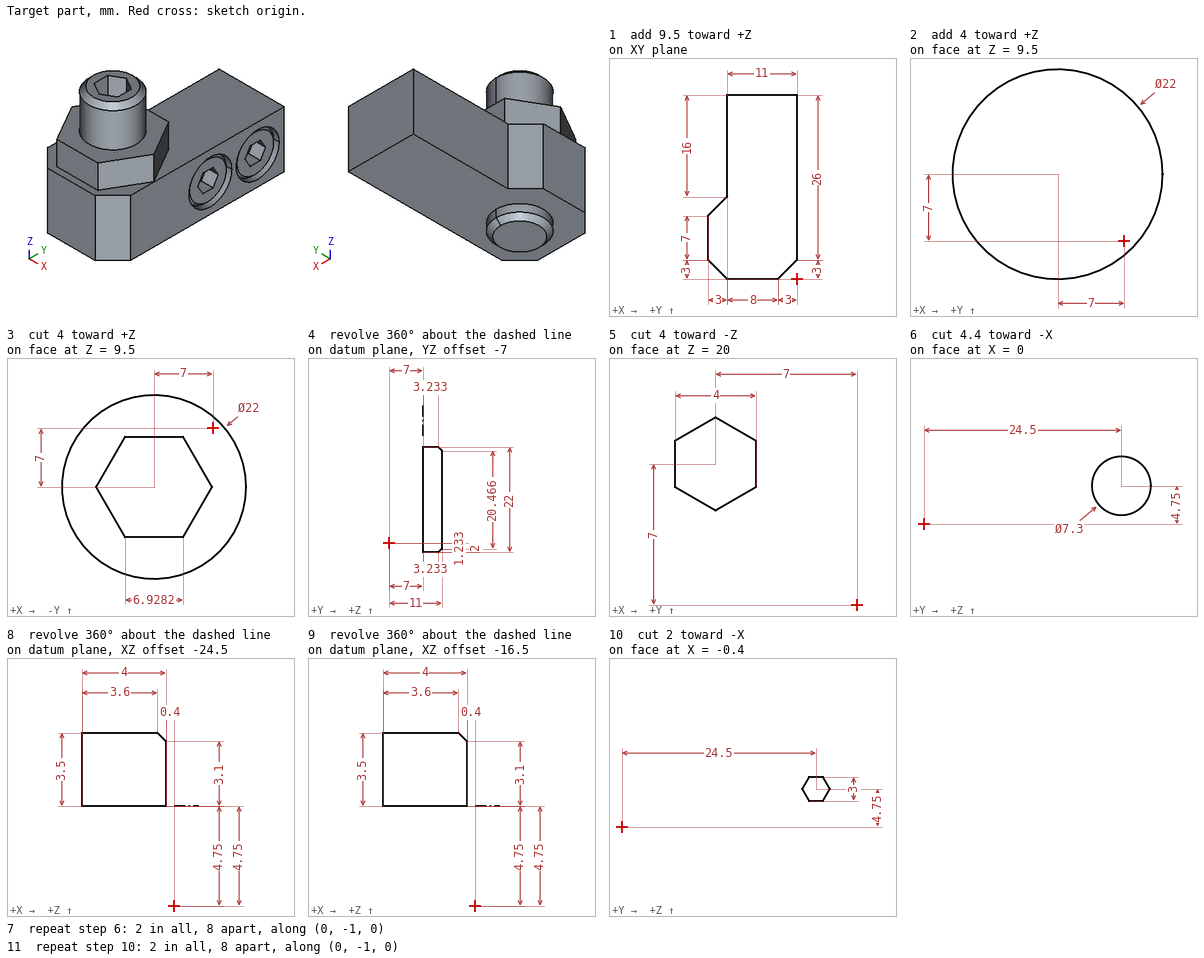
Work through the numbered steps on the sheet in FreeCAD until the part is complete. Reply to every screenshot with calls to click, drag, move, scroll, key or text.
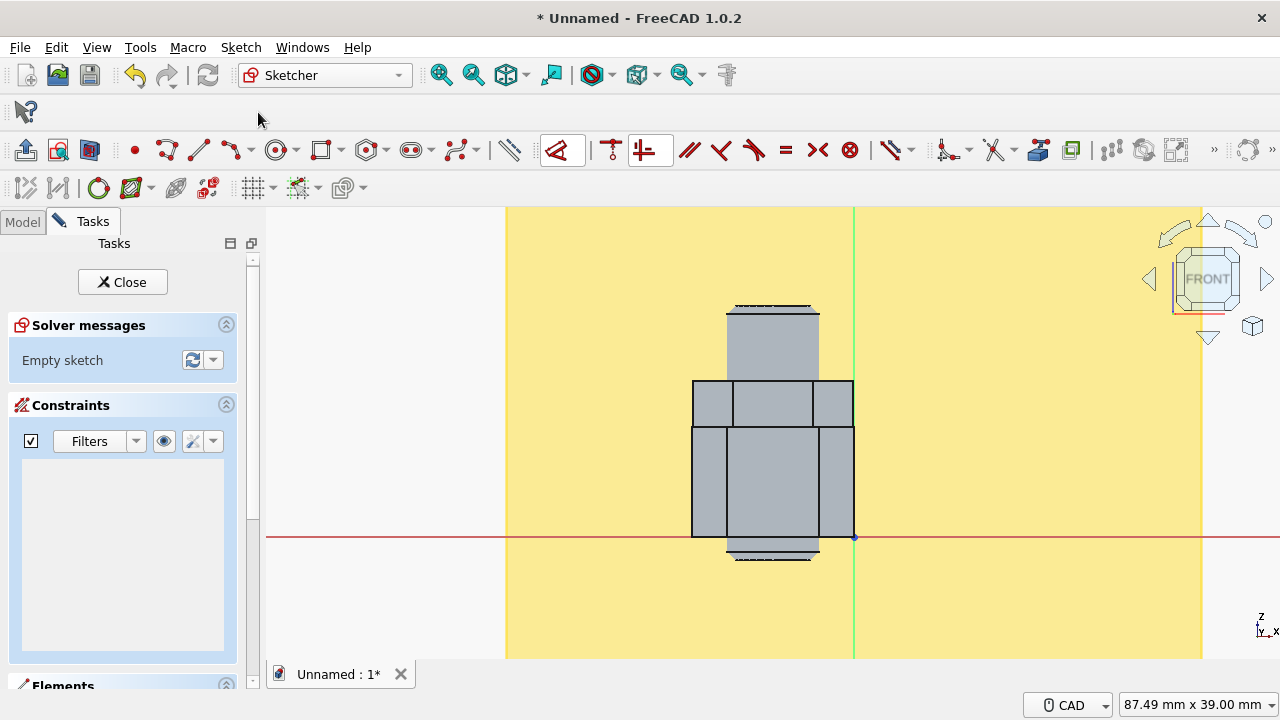
key(q)
key(s)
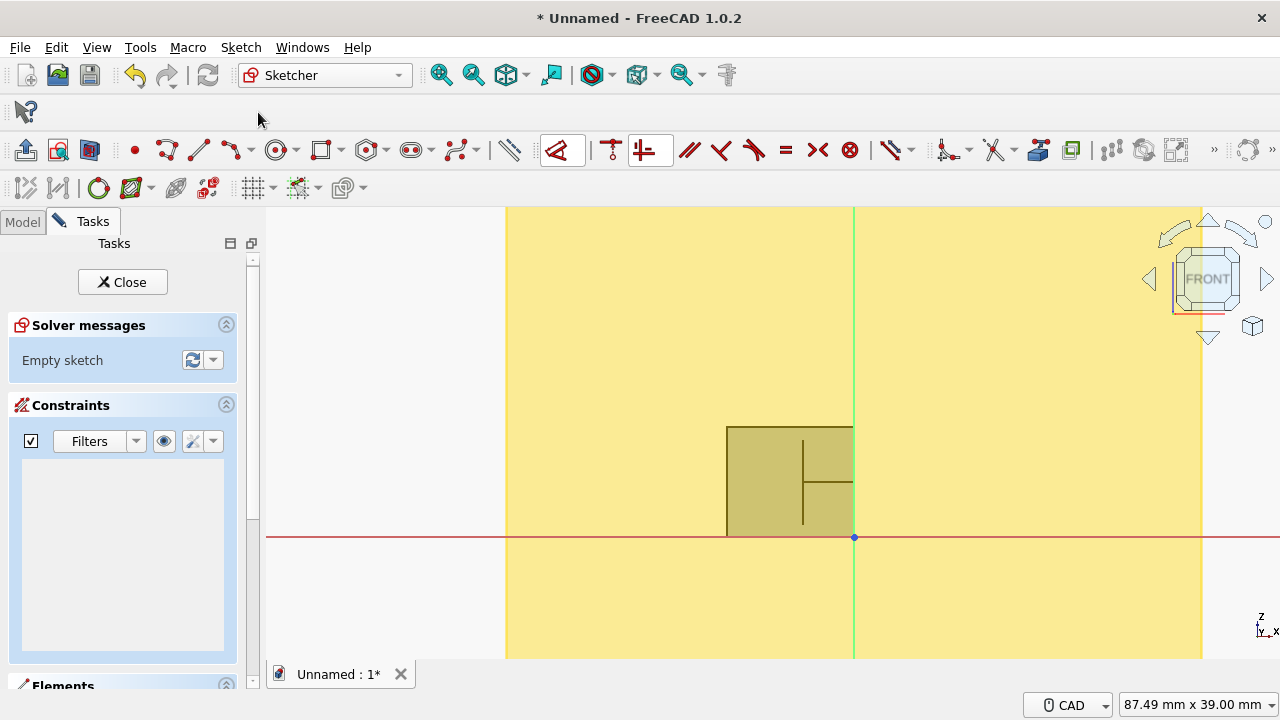
scroll(912, 522, up, 5)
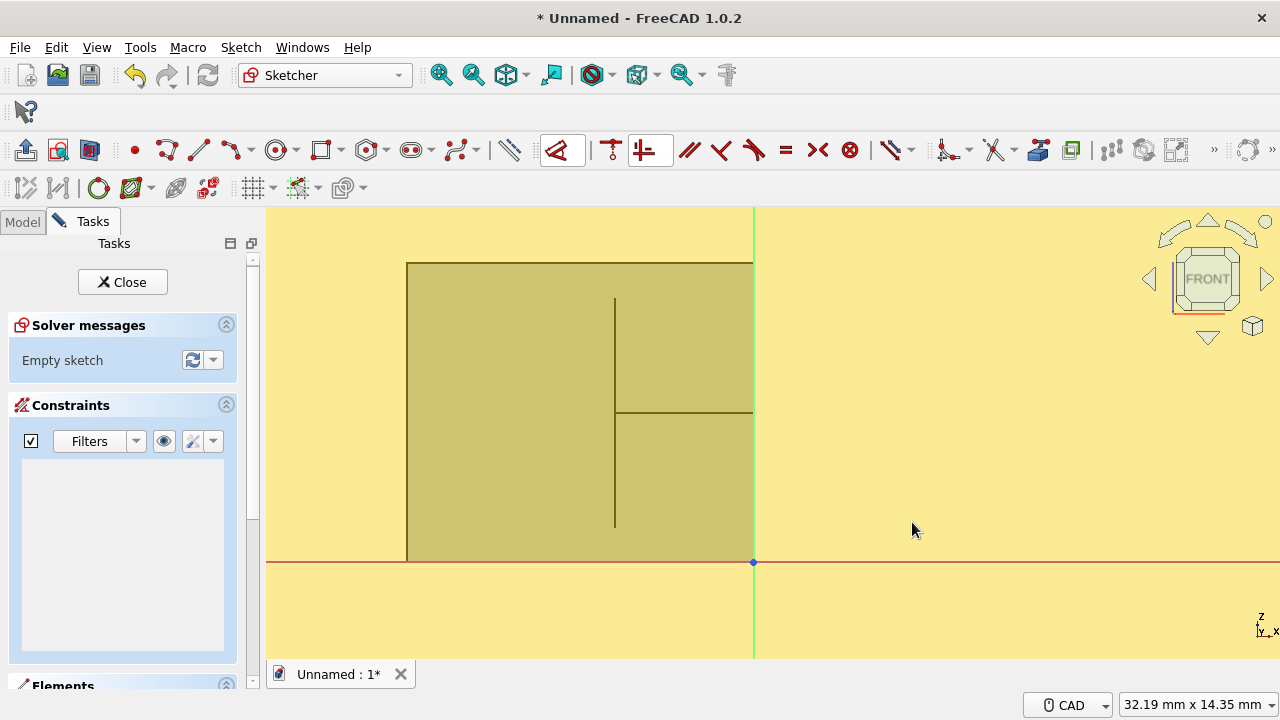
key(g)
key(m)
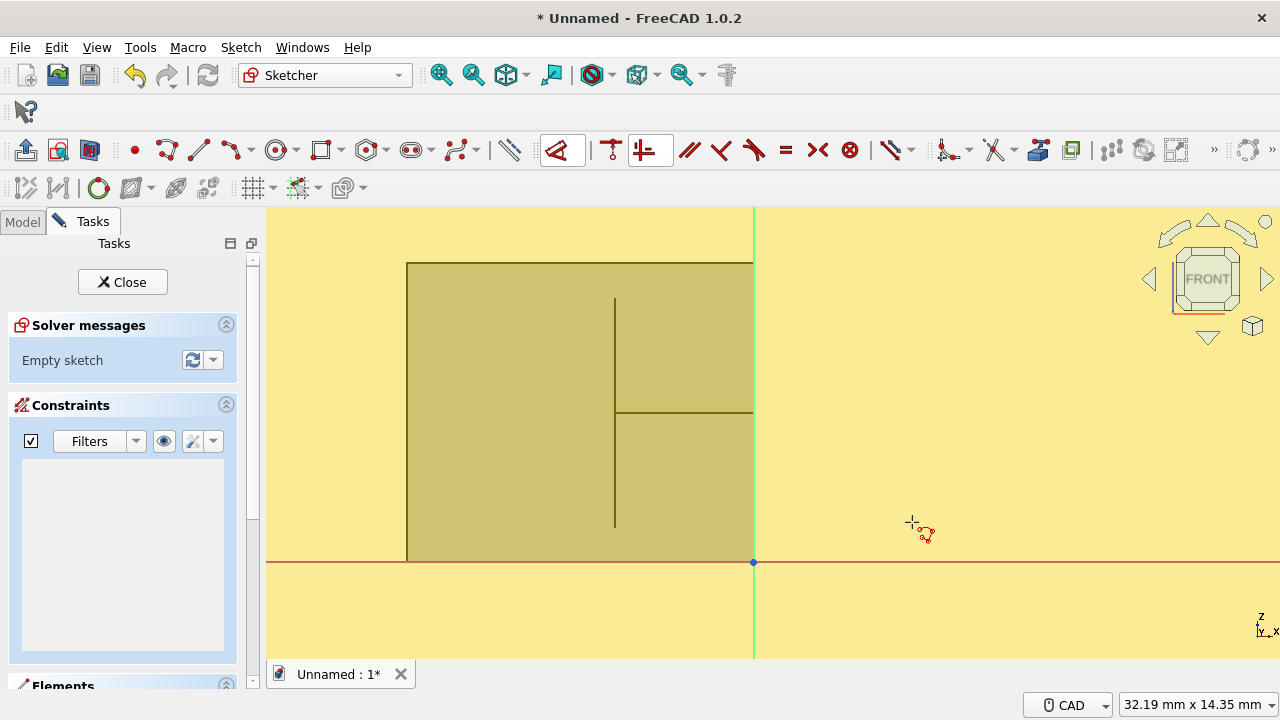
scroll(741, 413, up, 2)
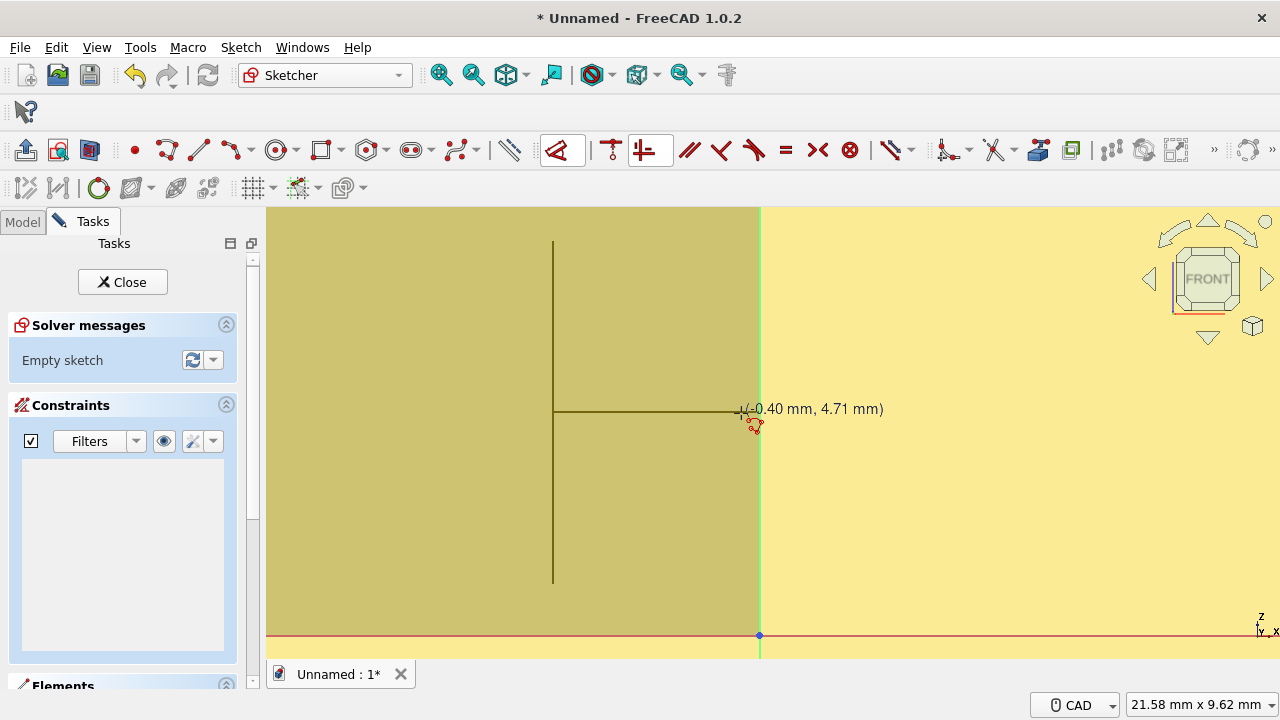
click(741, 412)
click(553, 412)
click(553, 248)
click(722, 248)
click(741, 267)
click(741, 413)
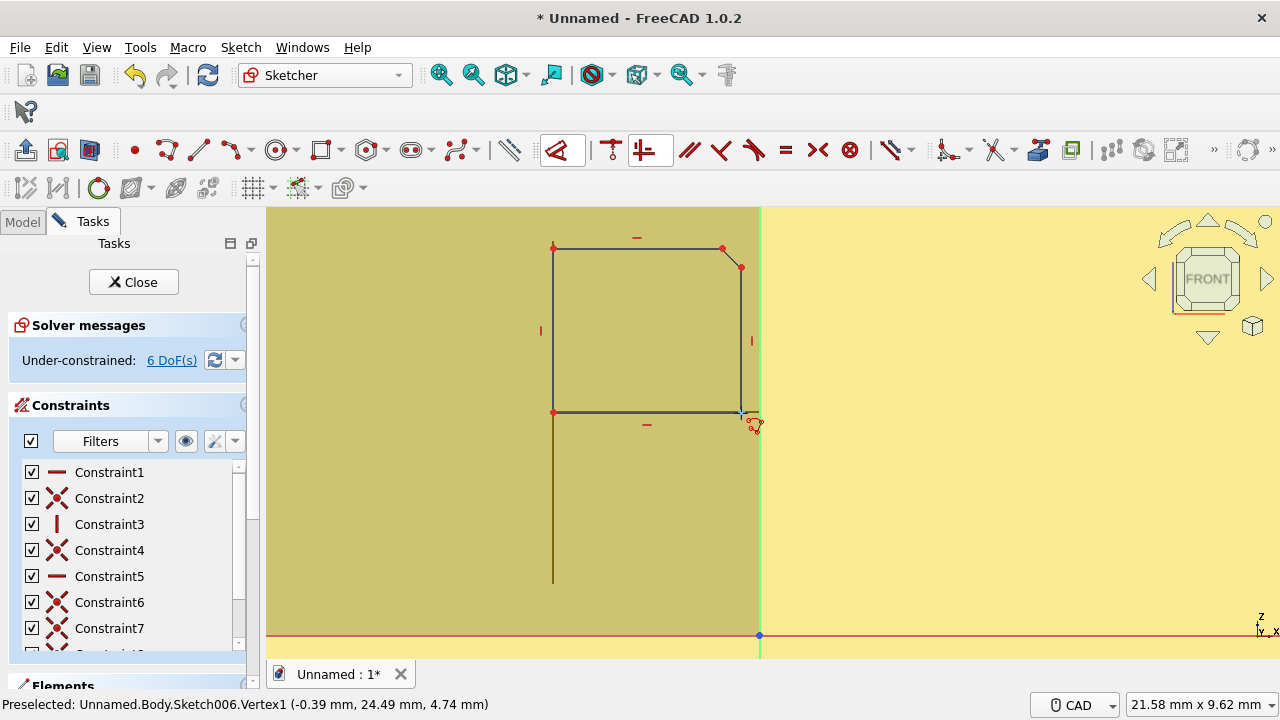
key(g)
key(l)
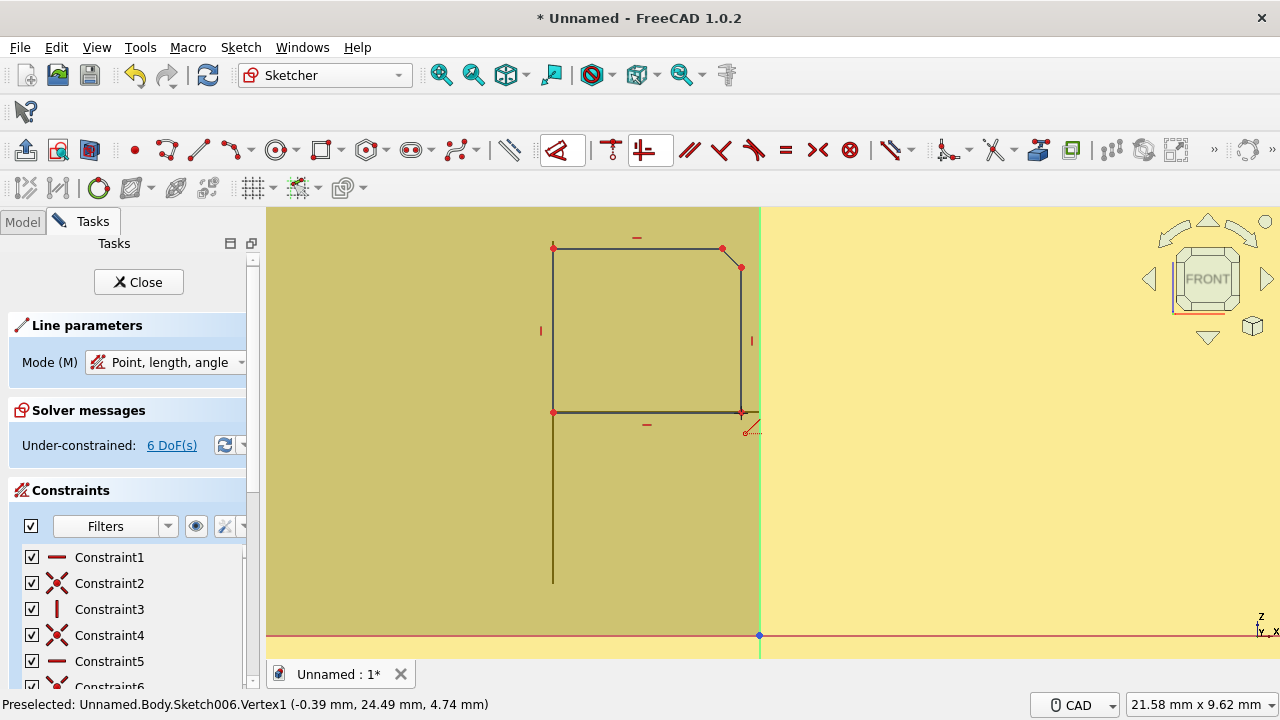
click(760, 412)
click(816, 412)
key(Escape)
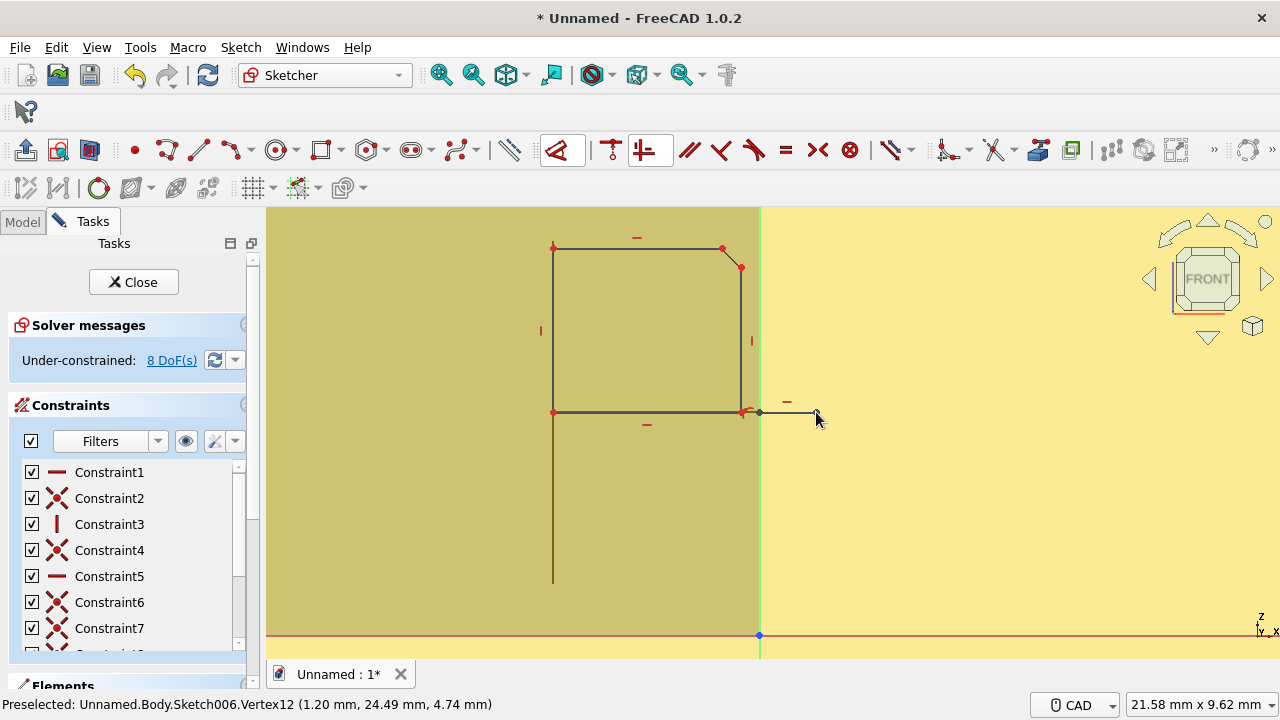
click(776, 413)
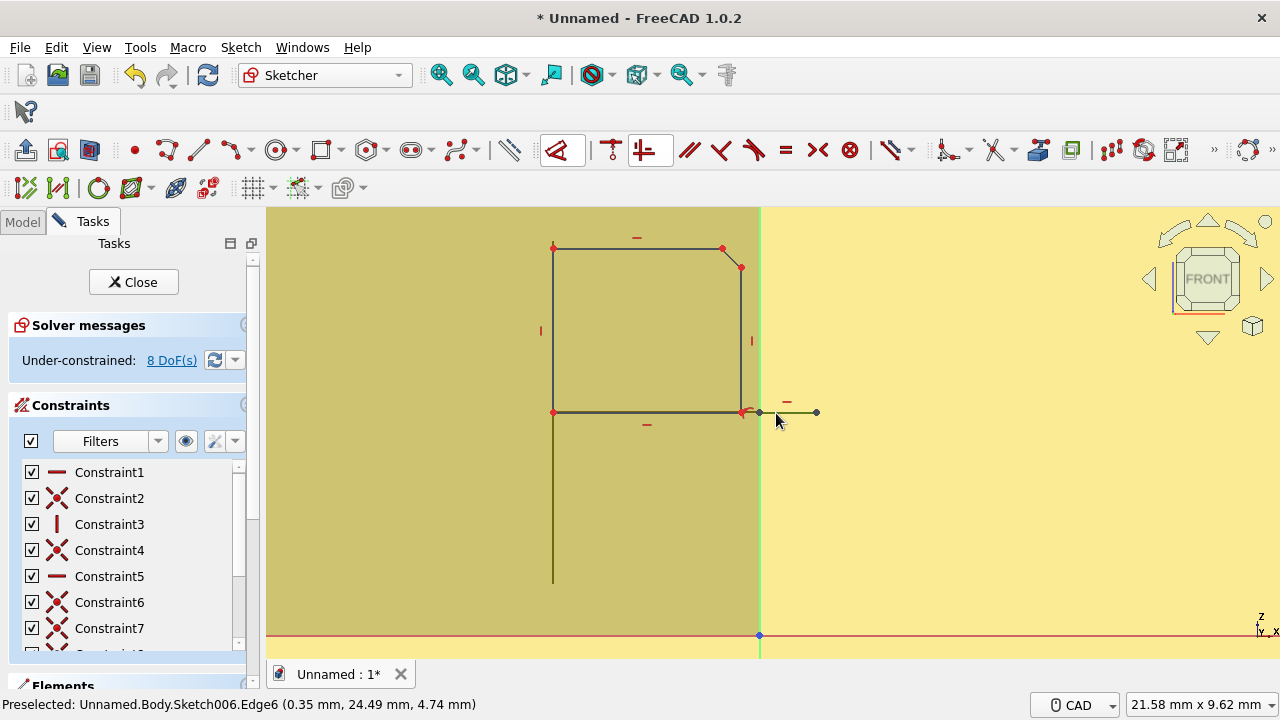
key(g)
key(n)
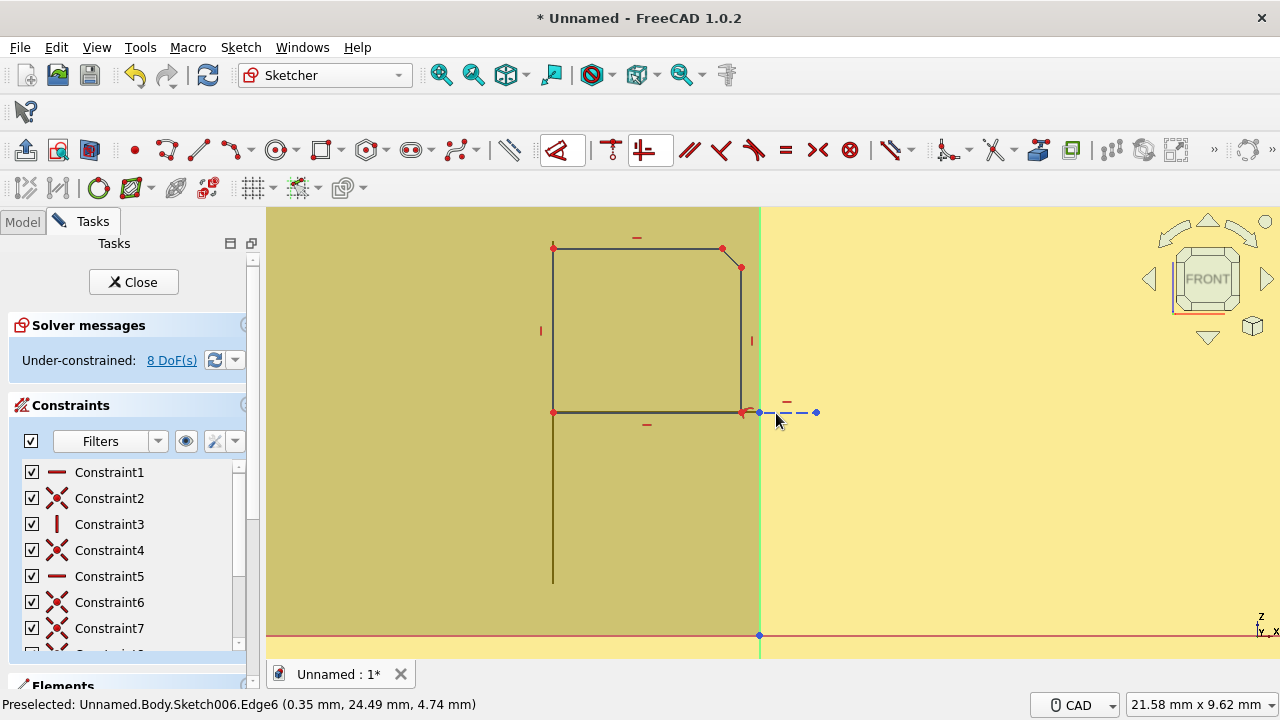
click(685, 413)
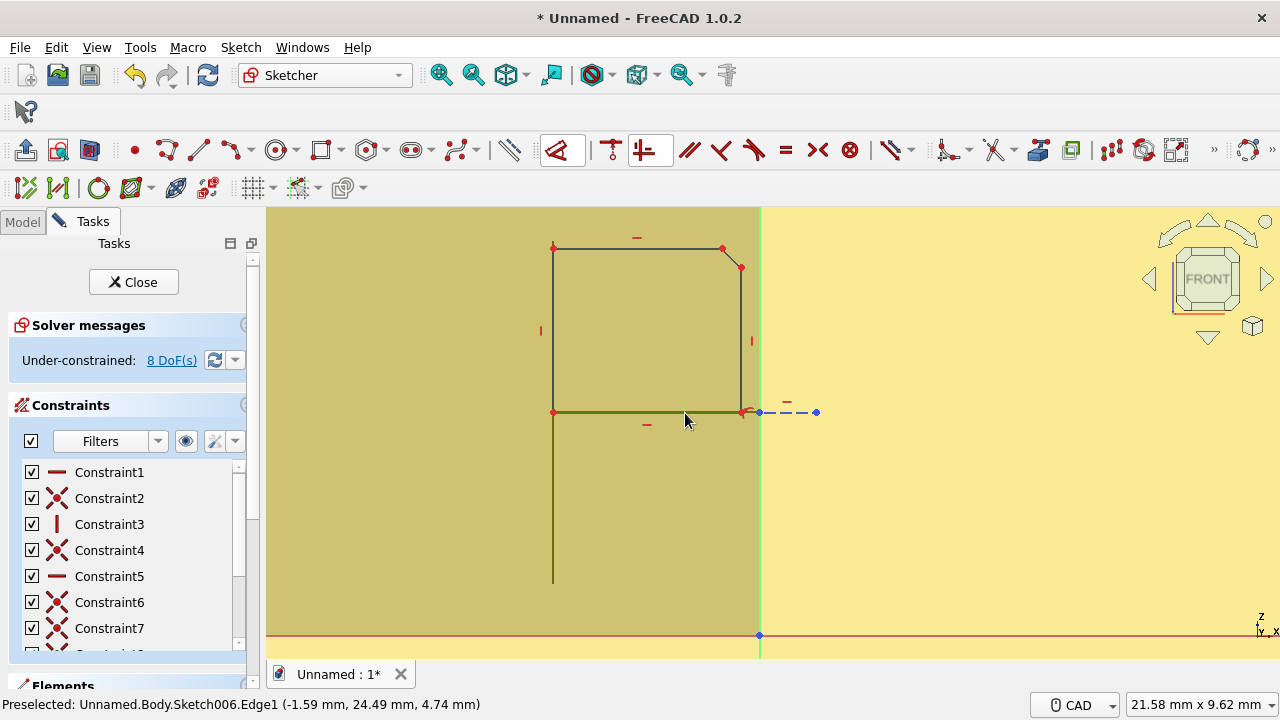
key(l)